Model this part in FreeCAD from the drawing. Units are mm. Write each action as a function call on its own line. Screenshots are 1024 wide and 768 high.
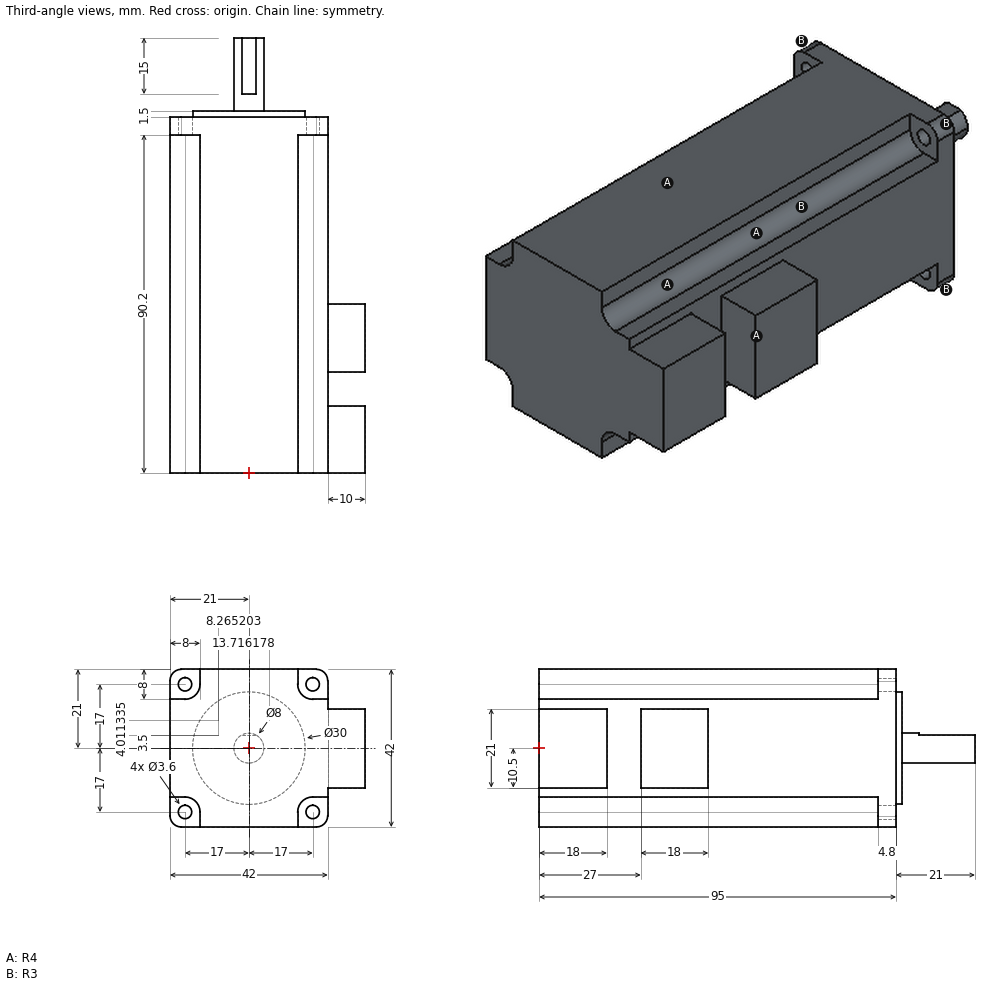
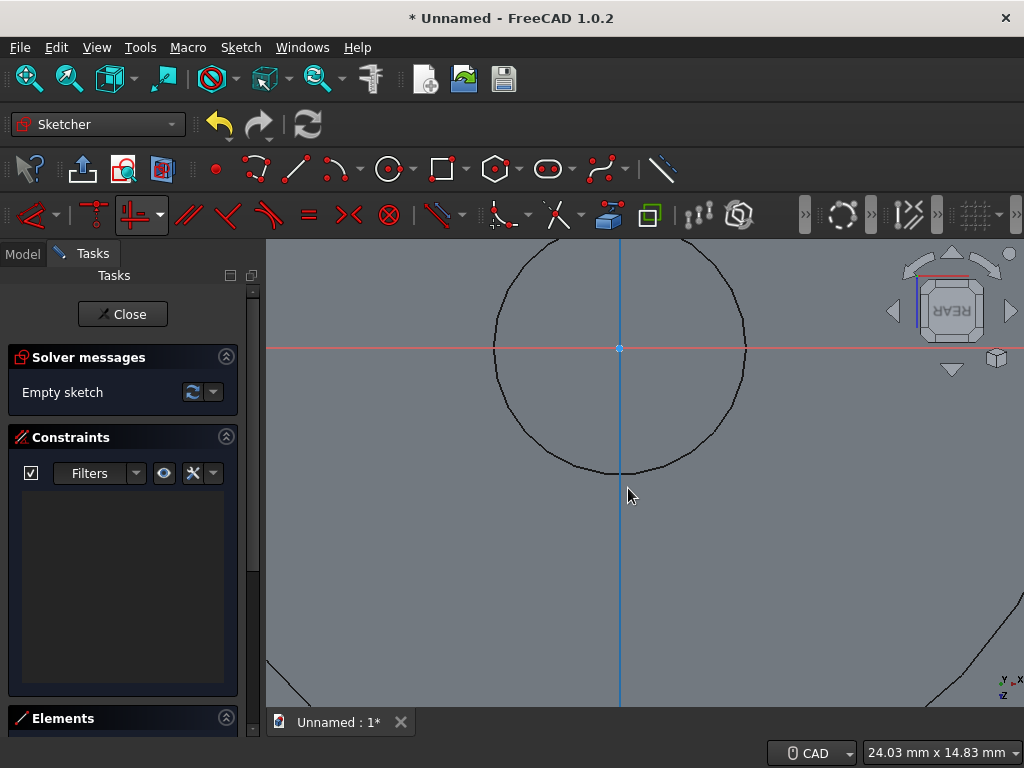
click(442, 170)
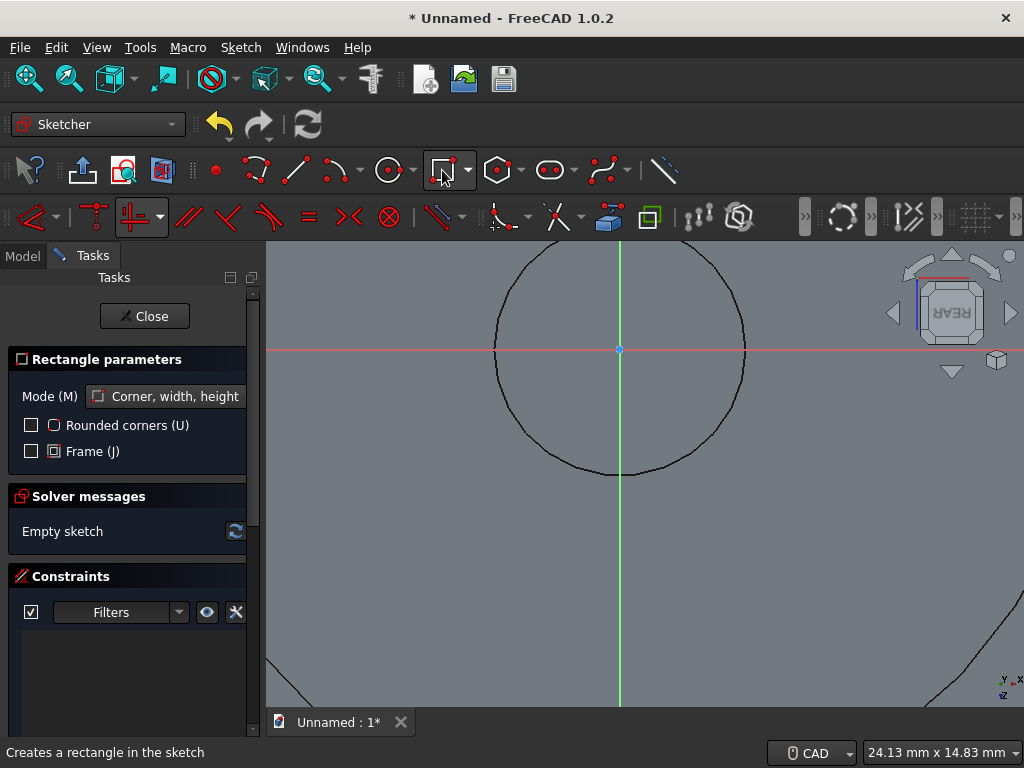
click(360, 460)
click(791, 586)
key(Escape)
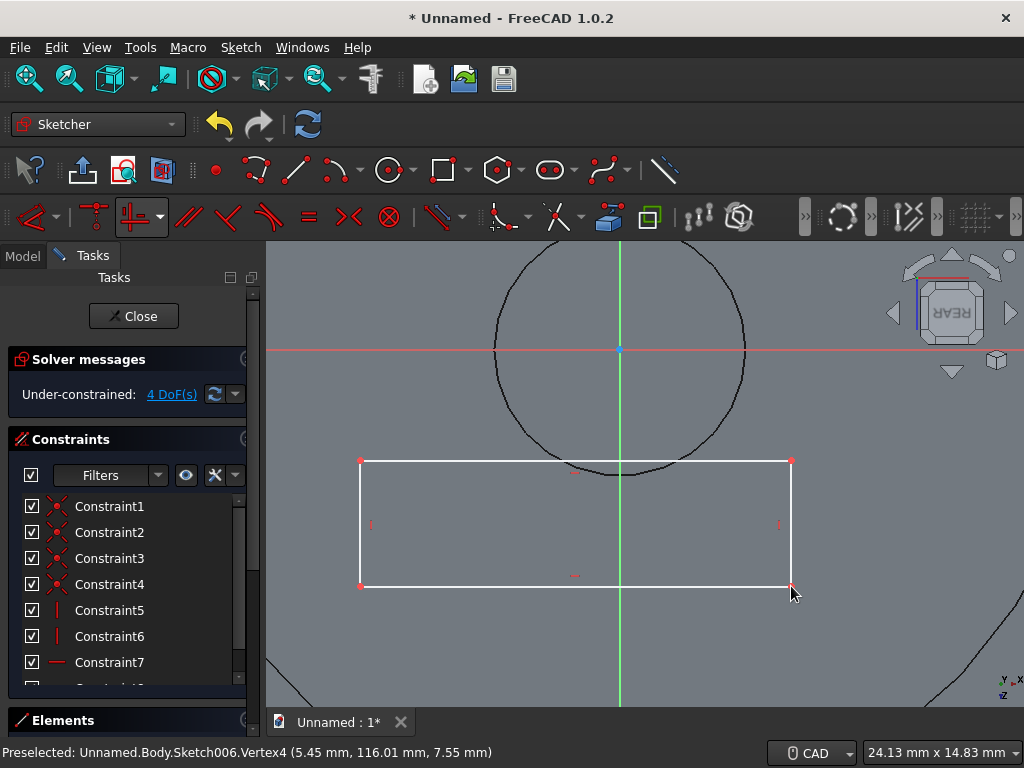
click(32, 218)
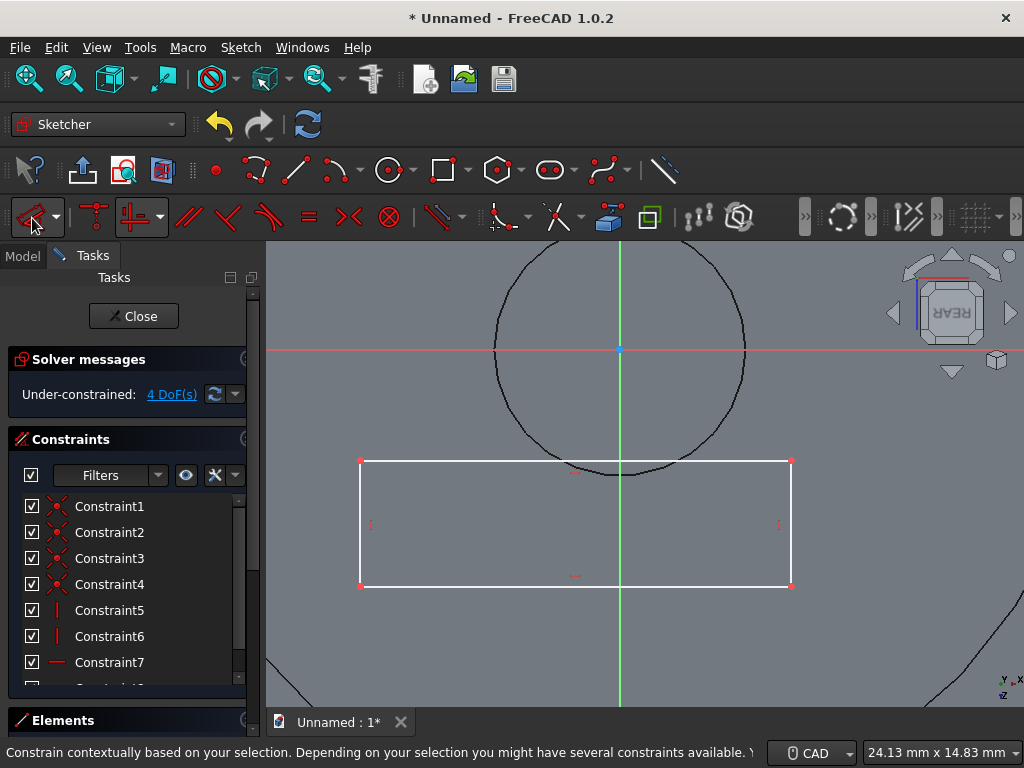
click(360, 461)
click(326, 405)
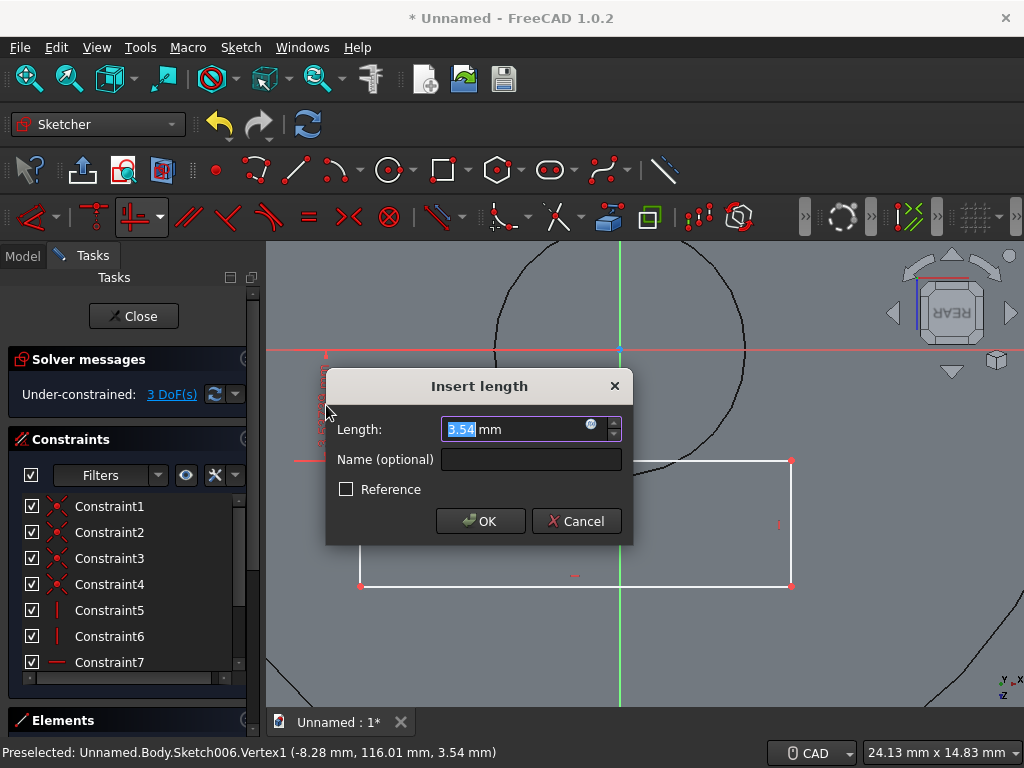
text(3.5)
key(Return)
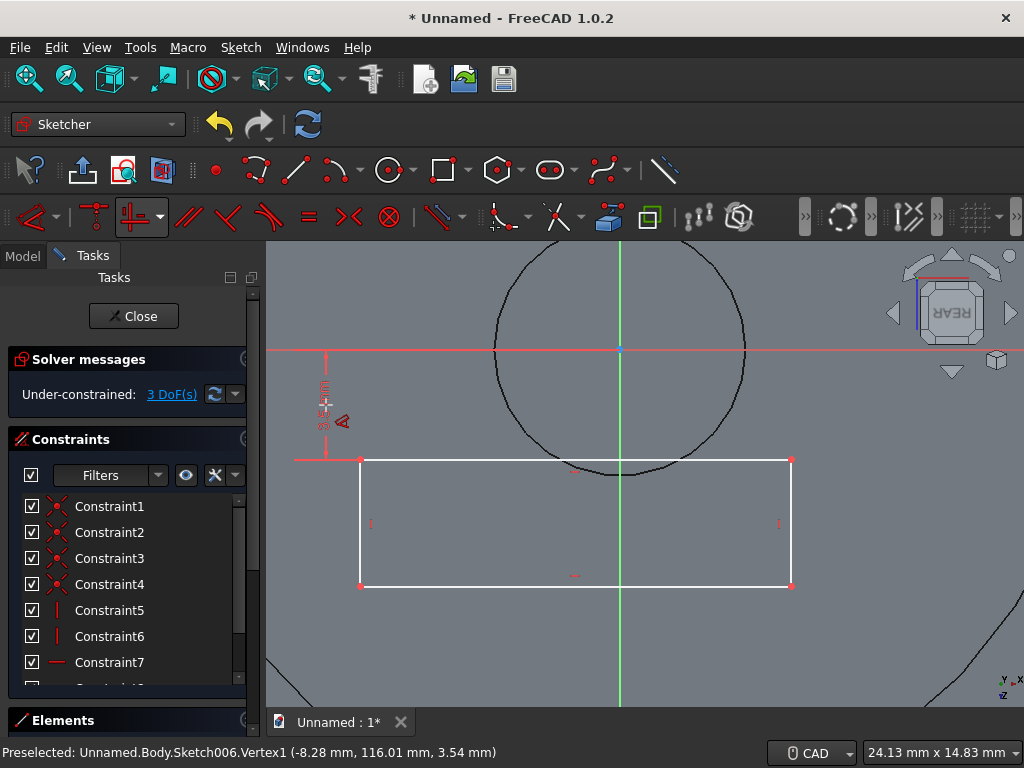
click(360, 498)
click(326, 523)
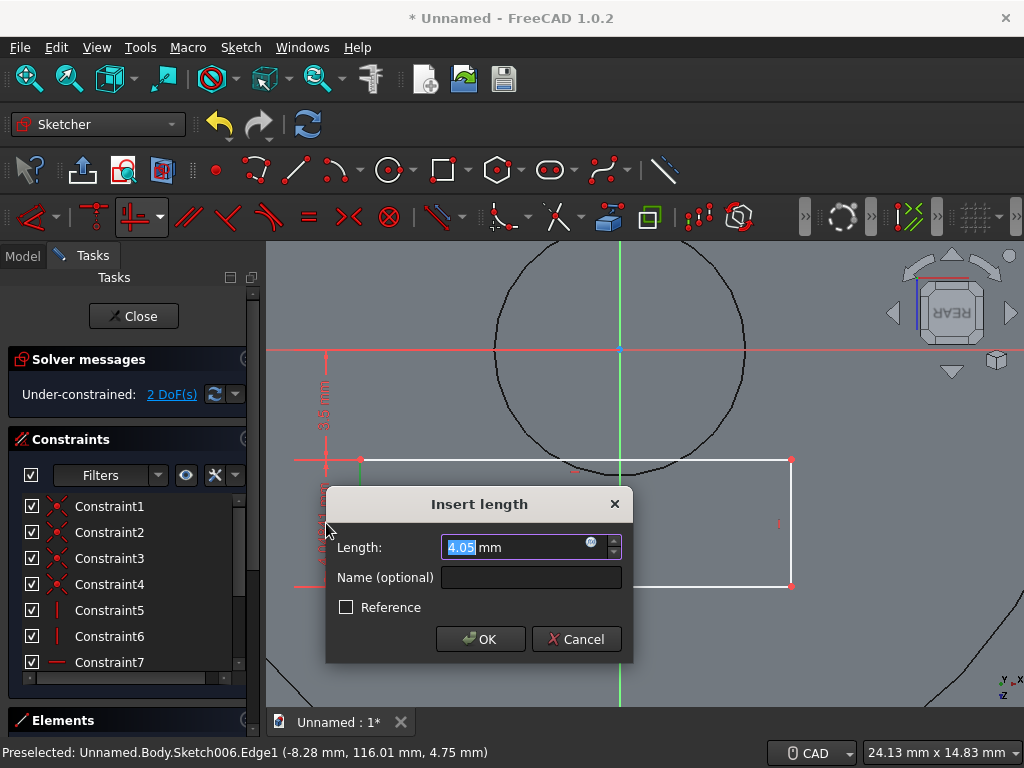
text(4.011335)
key(Return)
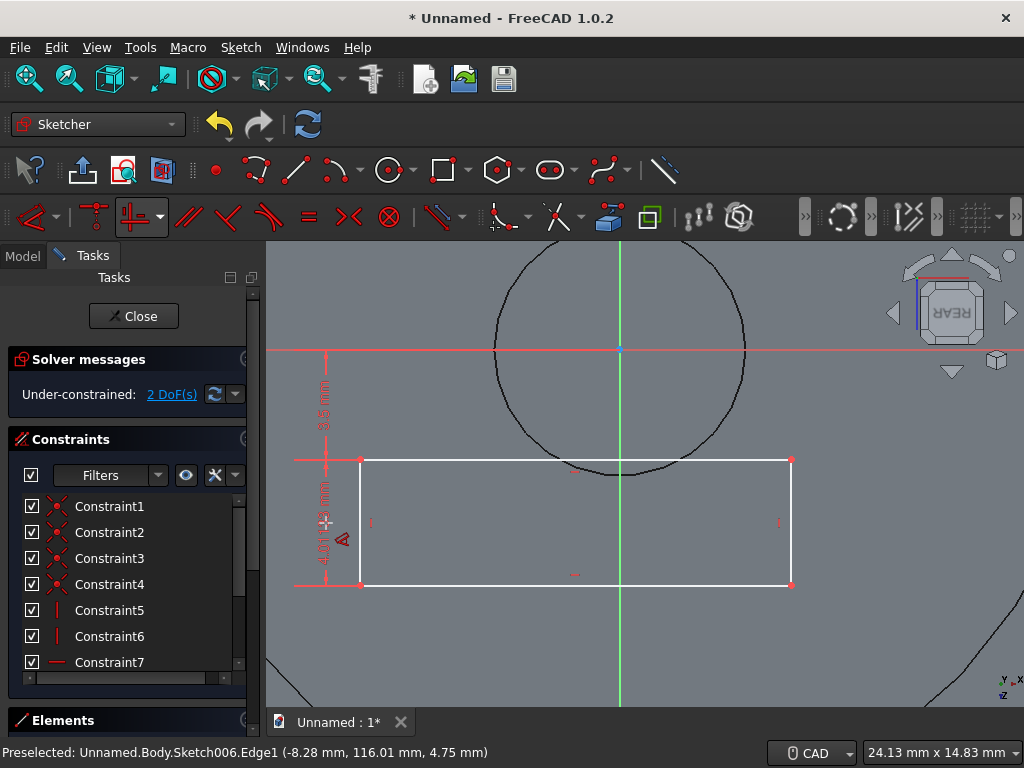
click(489, 586)
click(575, 620)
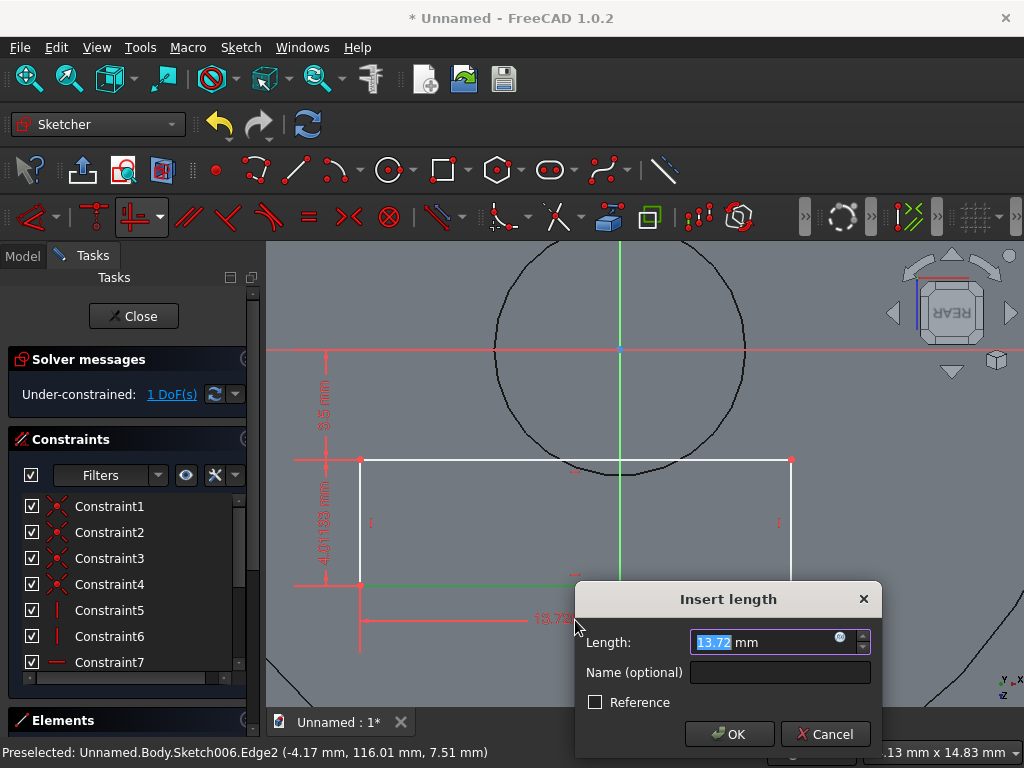
text(13.716178)
key(Return)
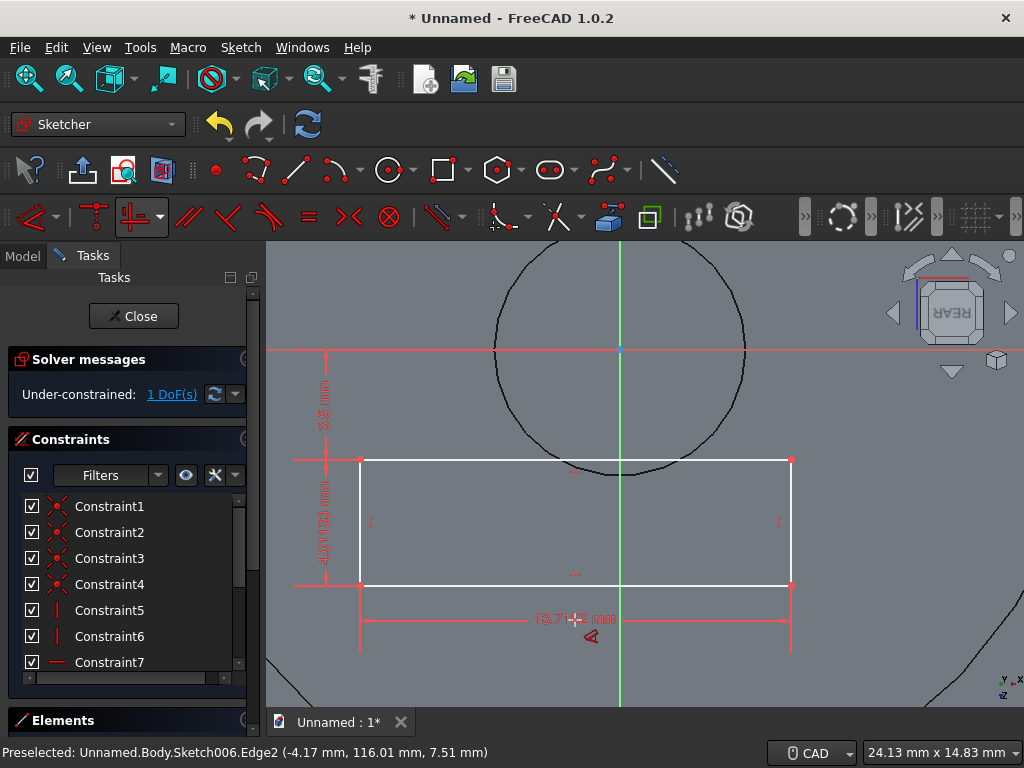
click(360, 460)
click(490, 316)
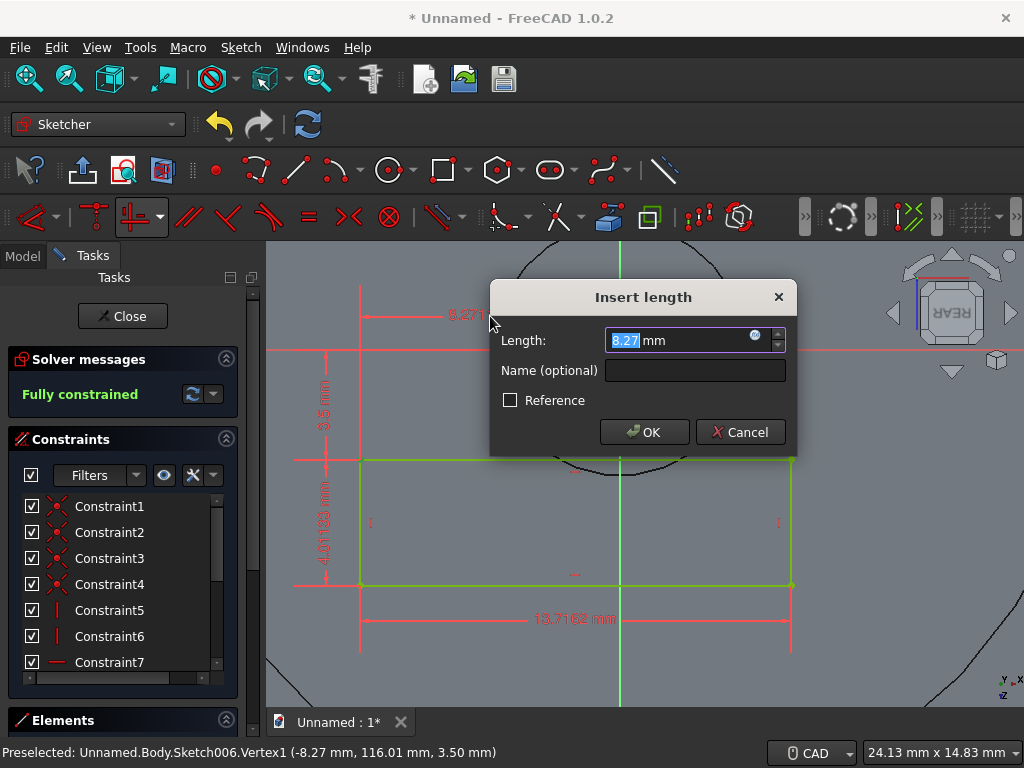
text(8.265203)
key(Return)
key(Escape)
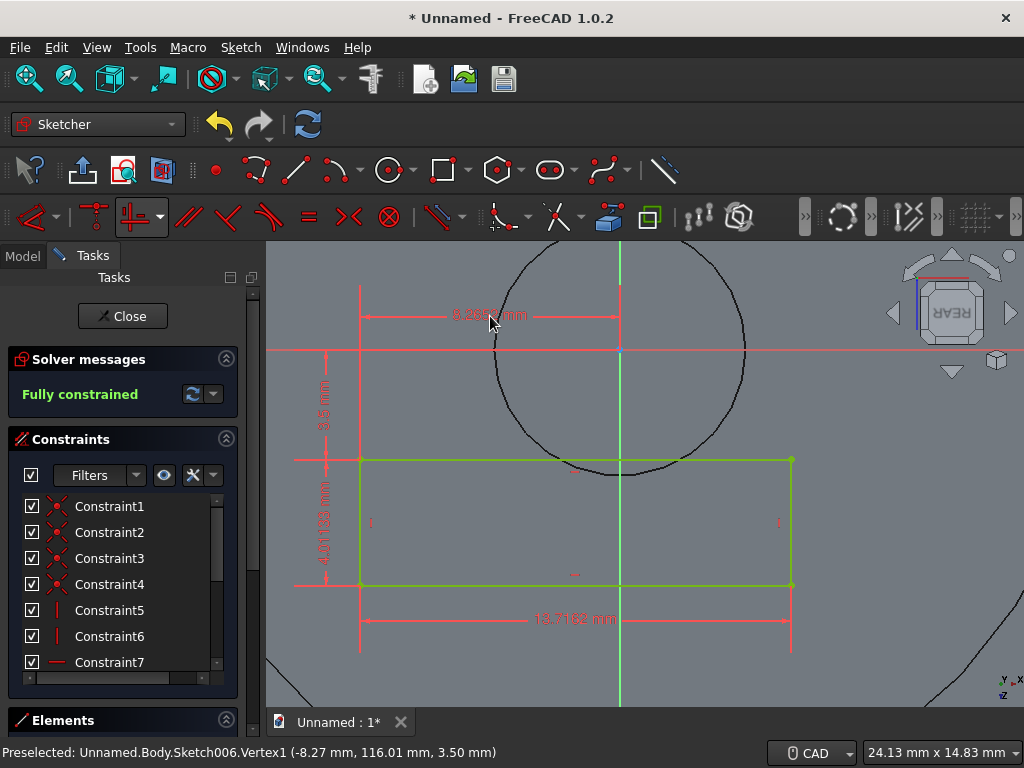
click(123, 316)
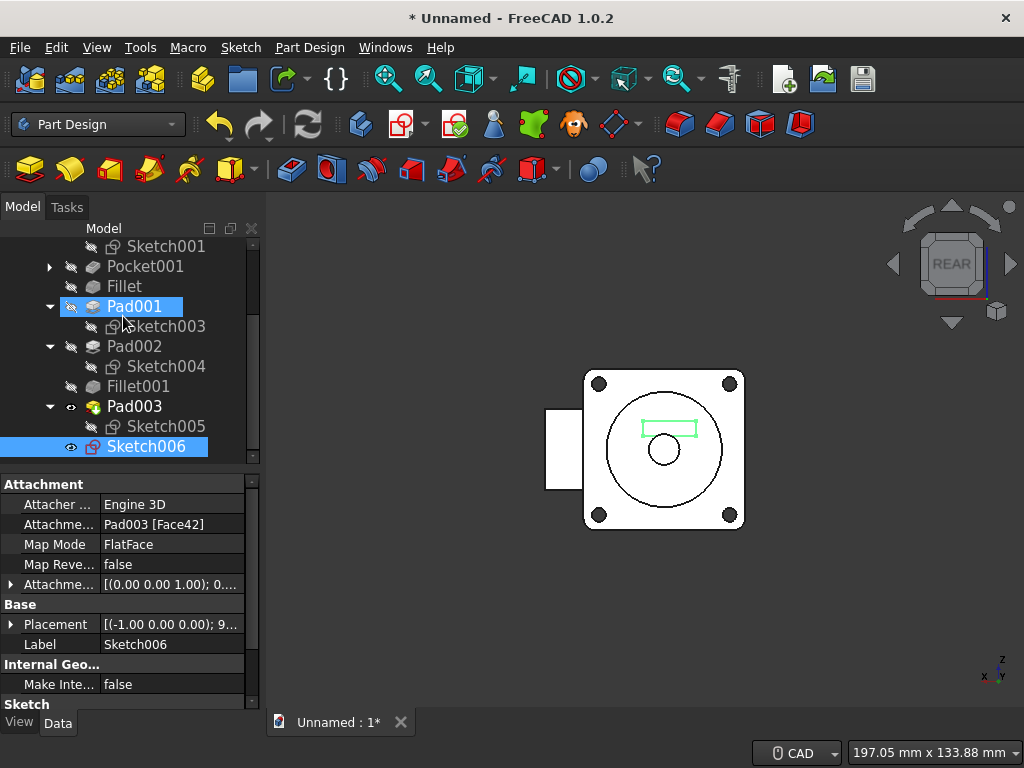
click(292, 170)